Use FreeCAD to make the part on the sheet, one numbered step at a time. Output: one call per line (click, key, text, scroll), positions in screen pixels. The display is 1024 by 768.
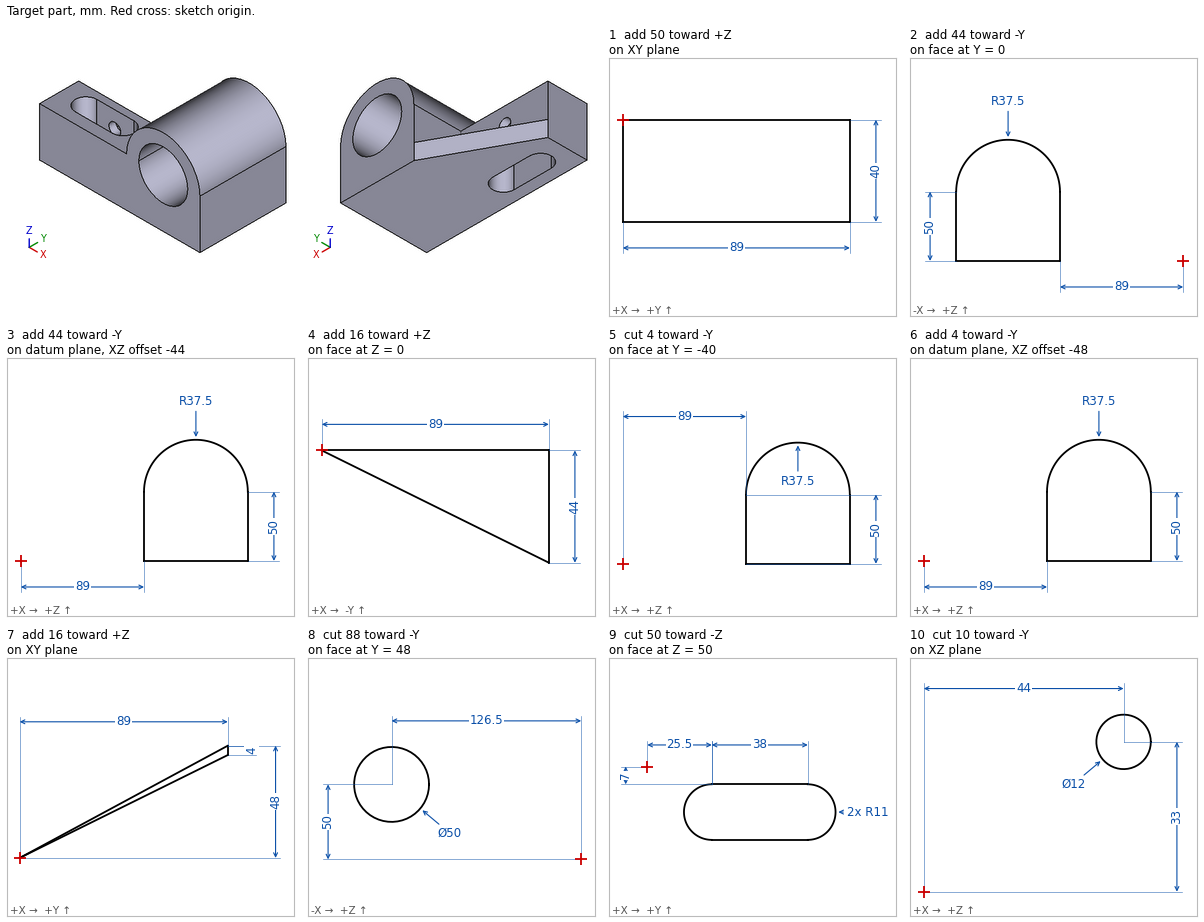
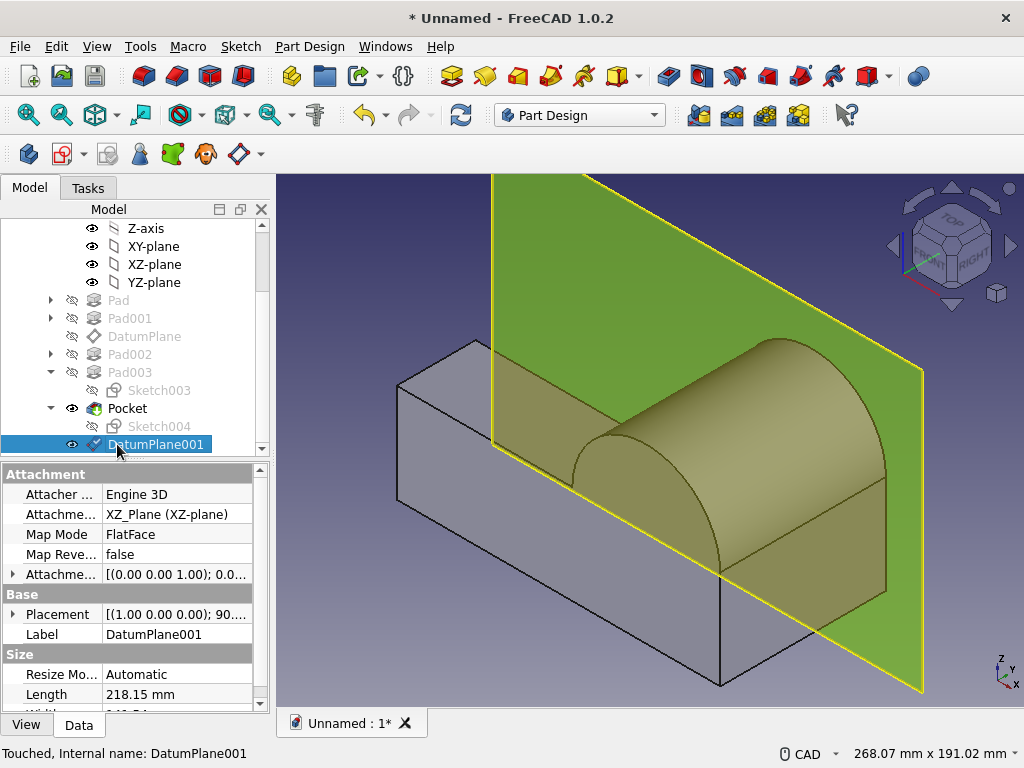
click(62, 154)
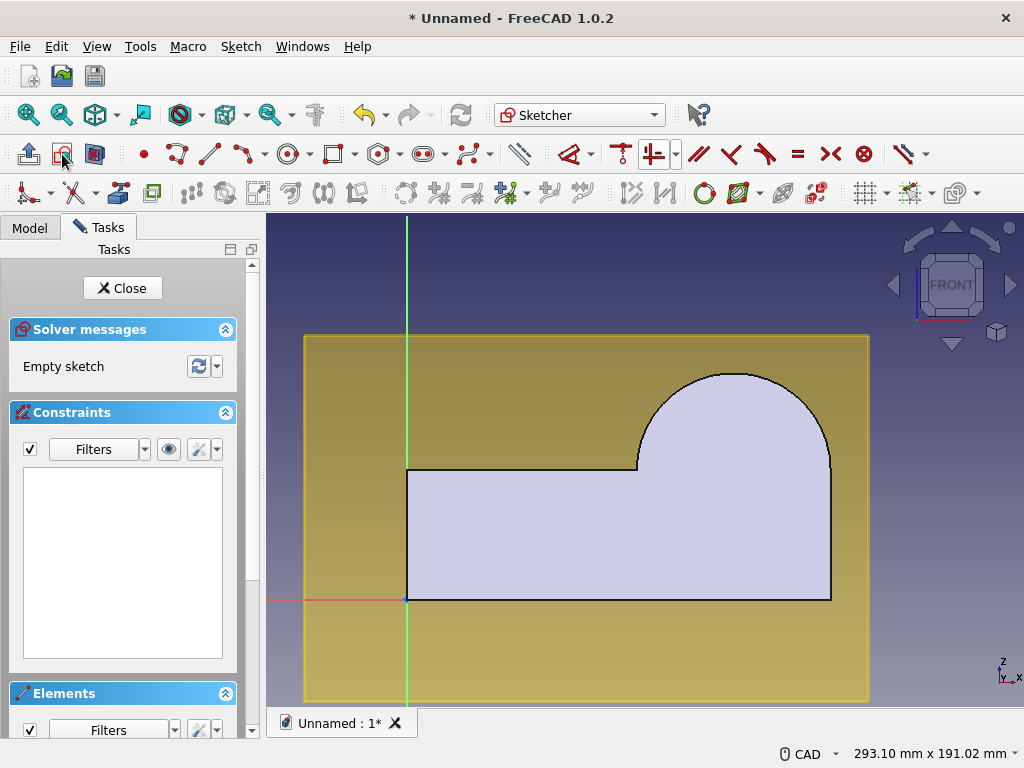
click(95, 154)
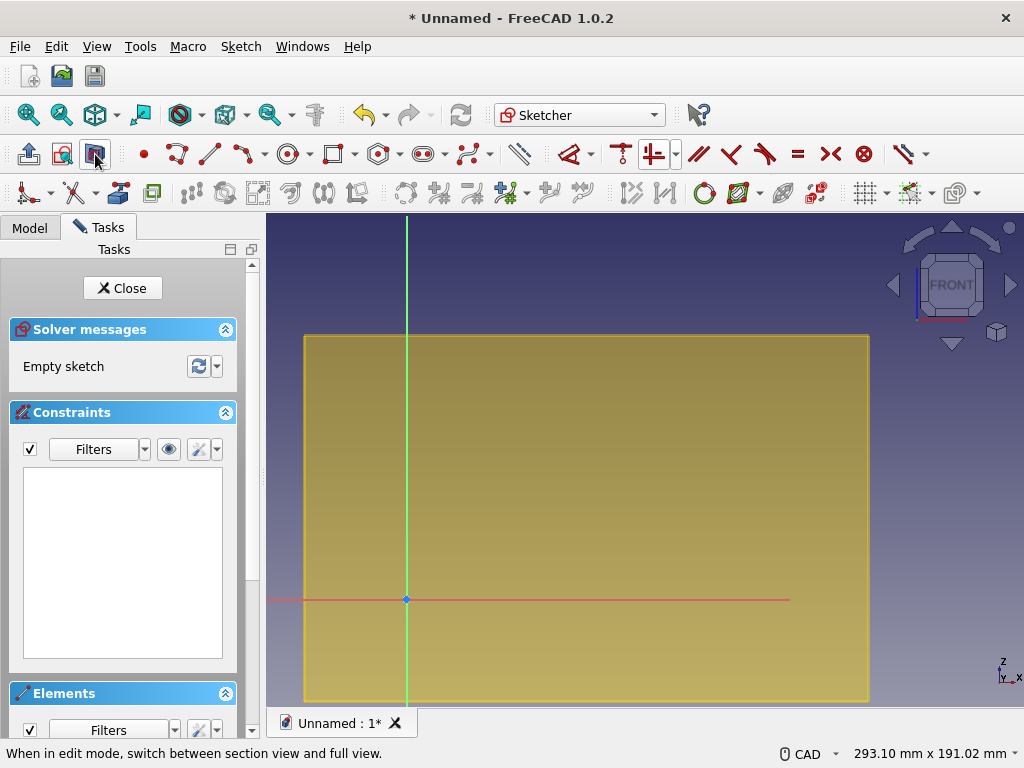
click(177, 154)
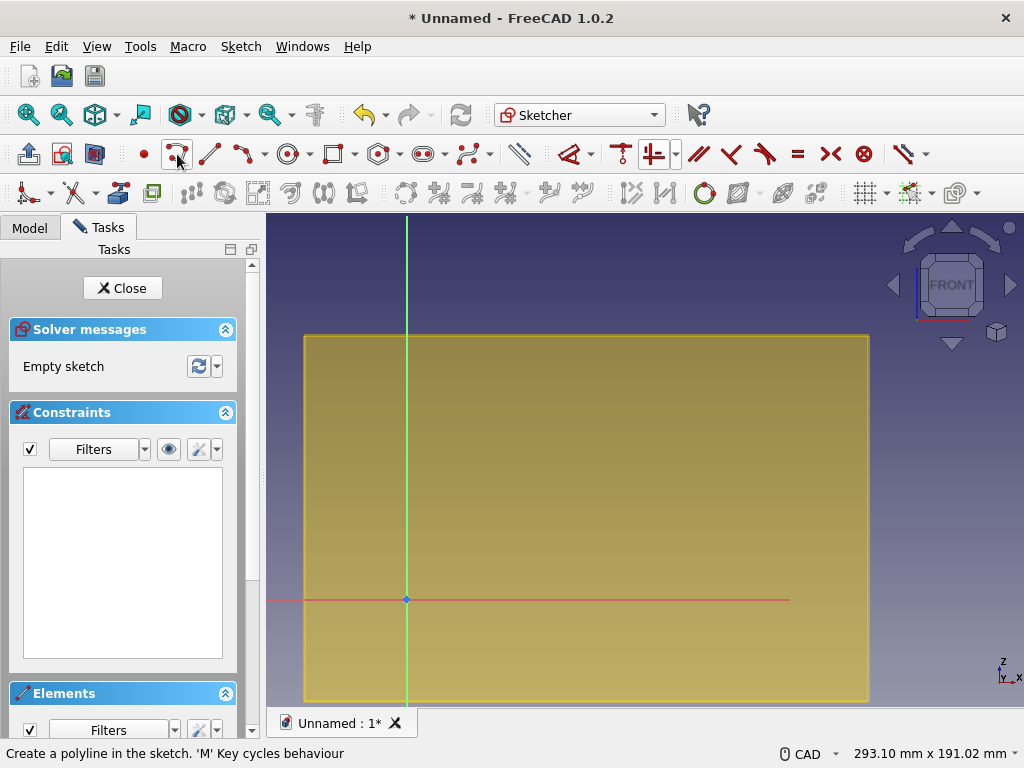
click(831, 470)
click(831, 600)
click(637, 591)
click(637, 470)
right_click(637, 470)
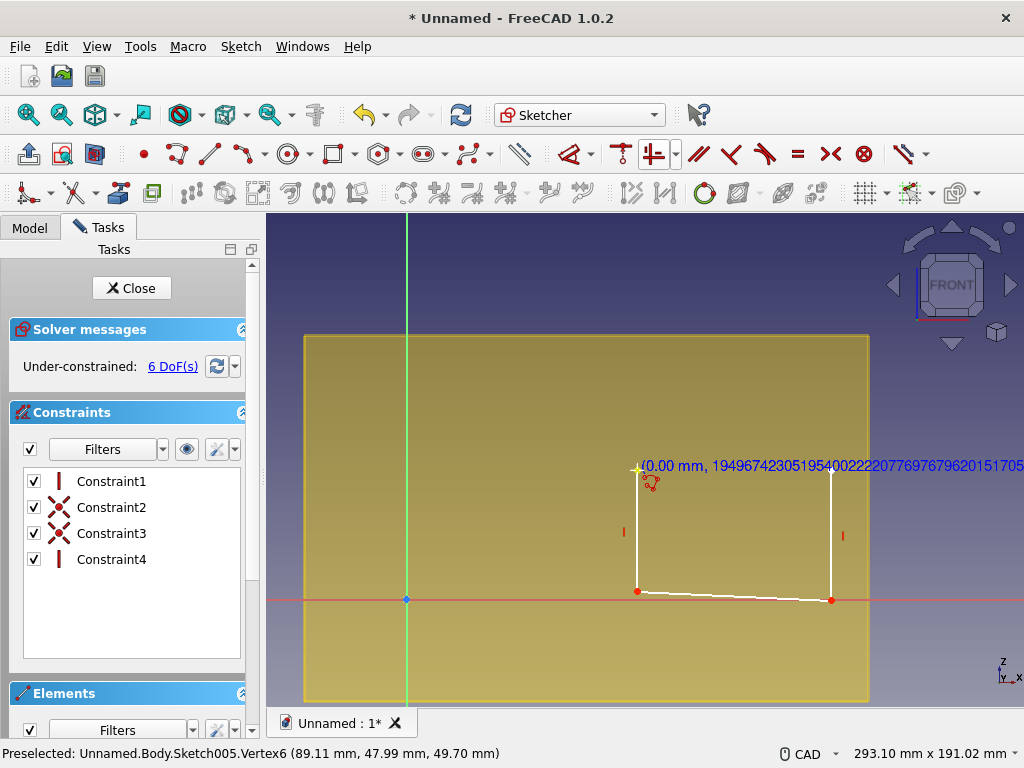
click(242, 154)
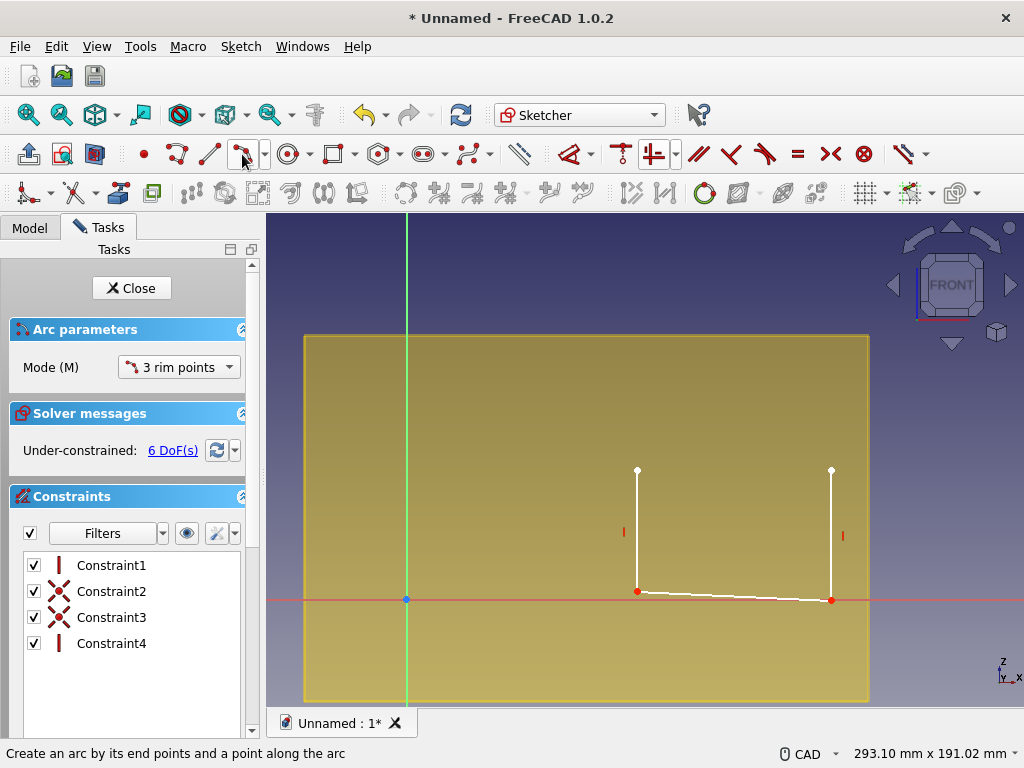
click(637, 471)
click(831, 471)
click(734, 373)
key(Escape)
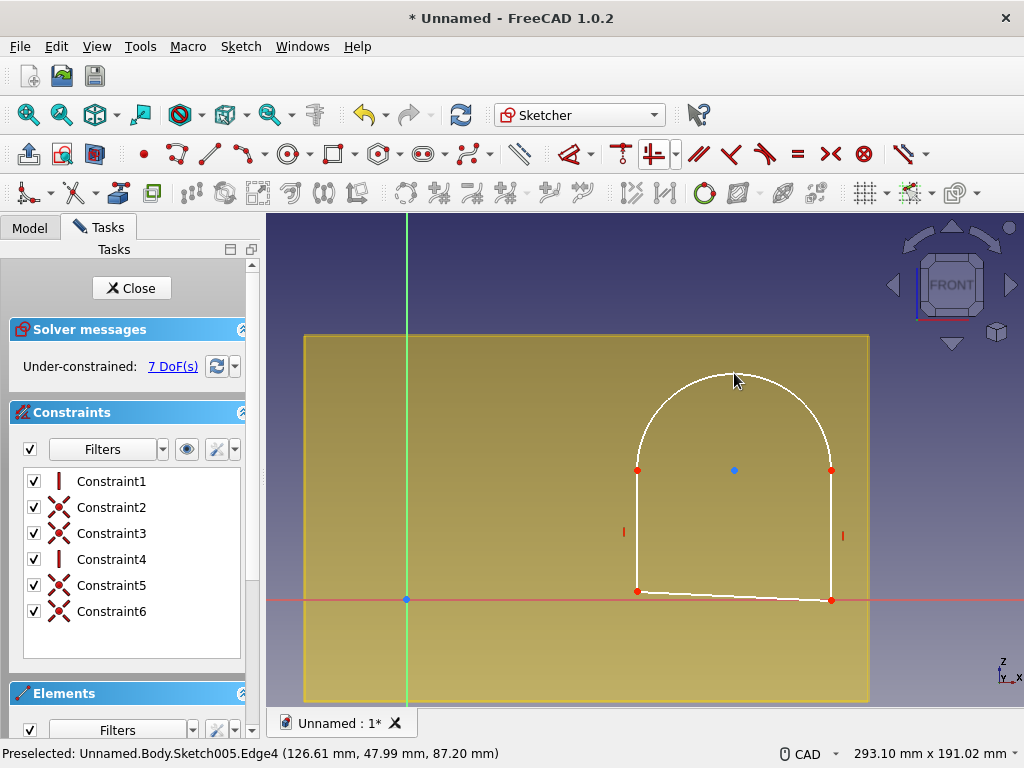
click(831, 510)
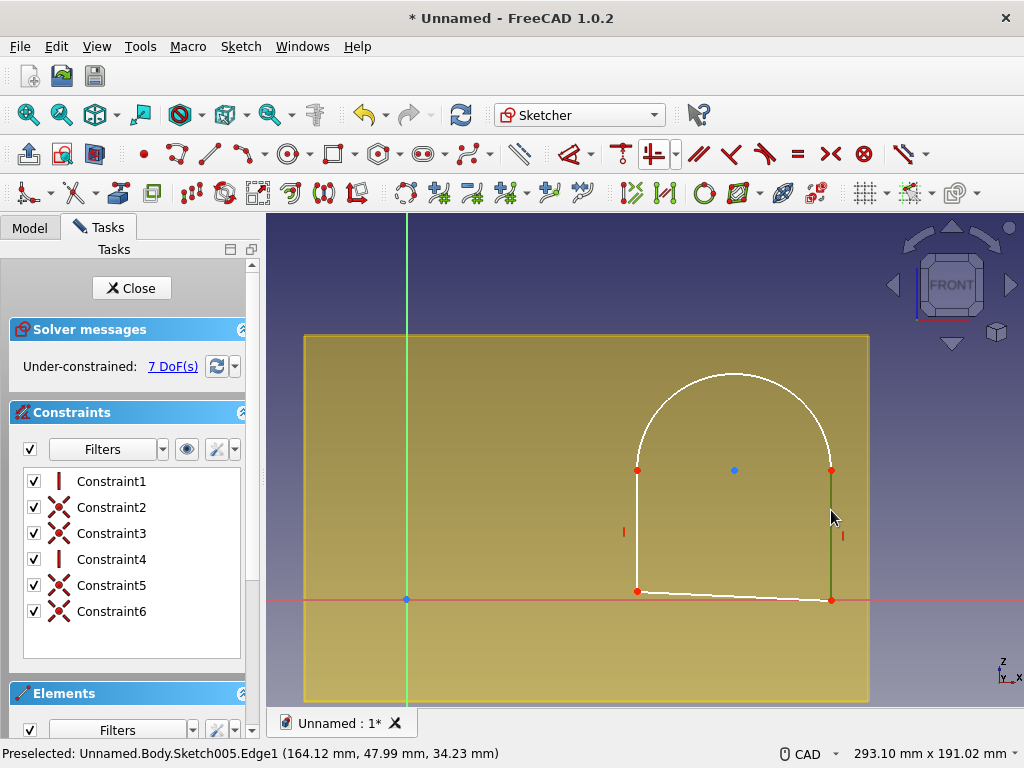
click(791, 393)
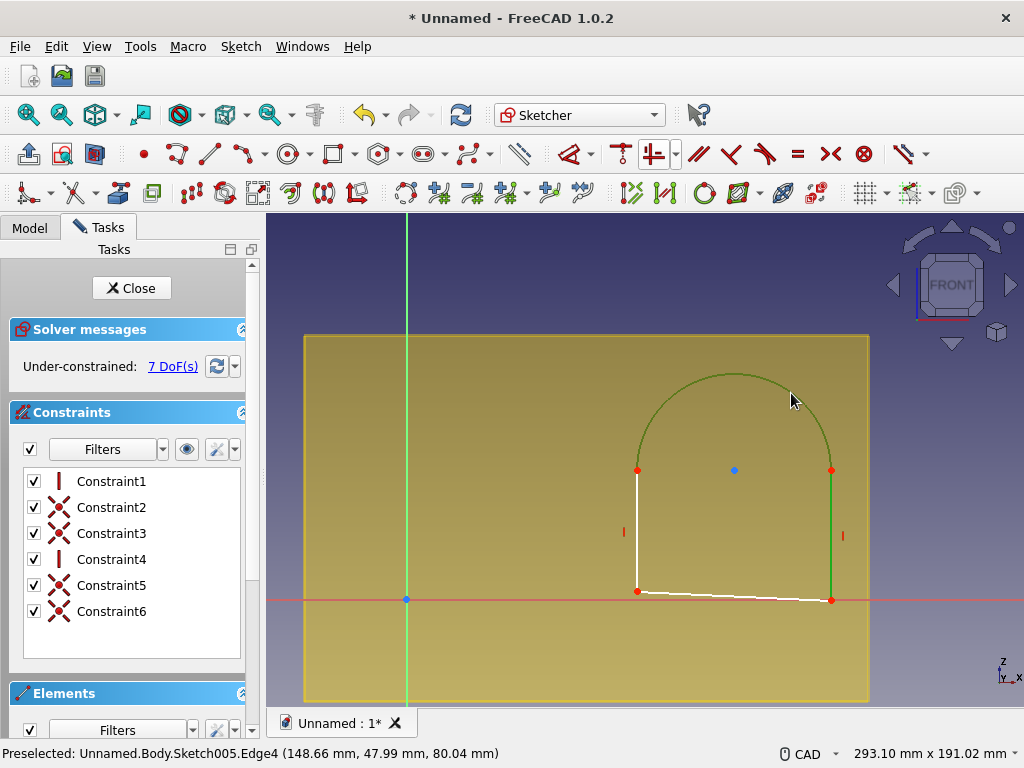
click(765, 154)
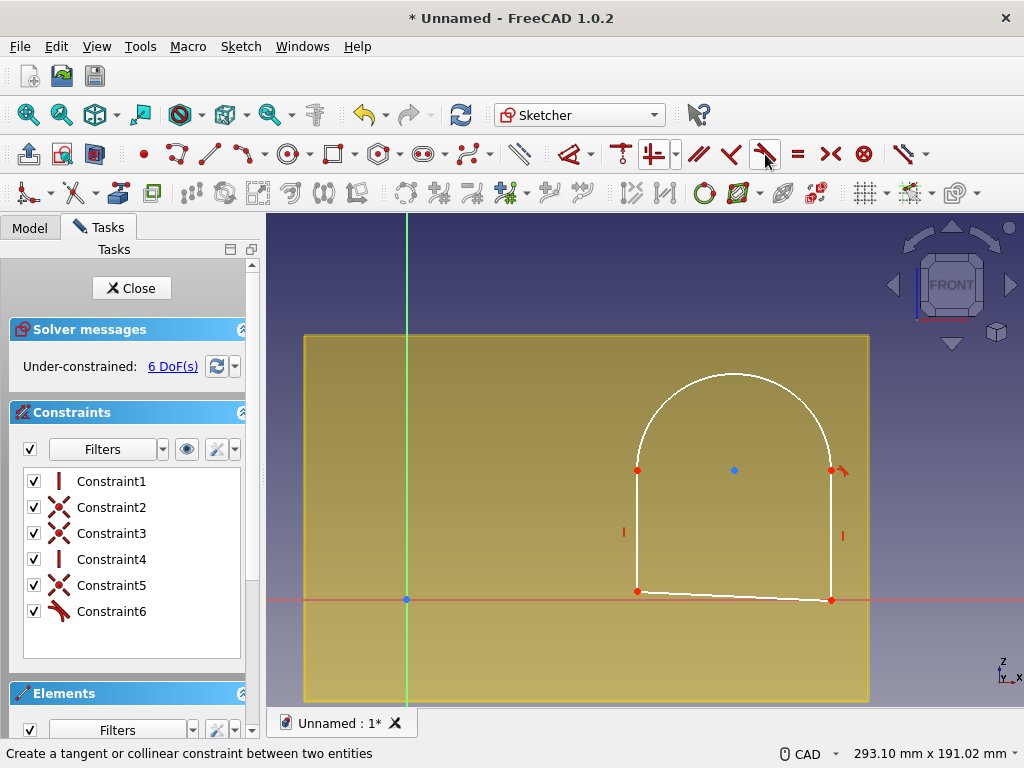
click(637, 556)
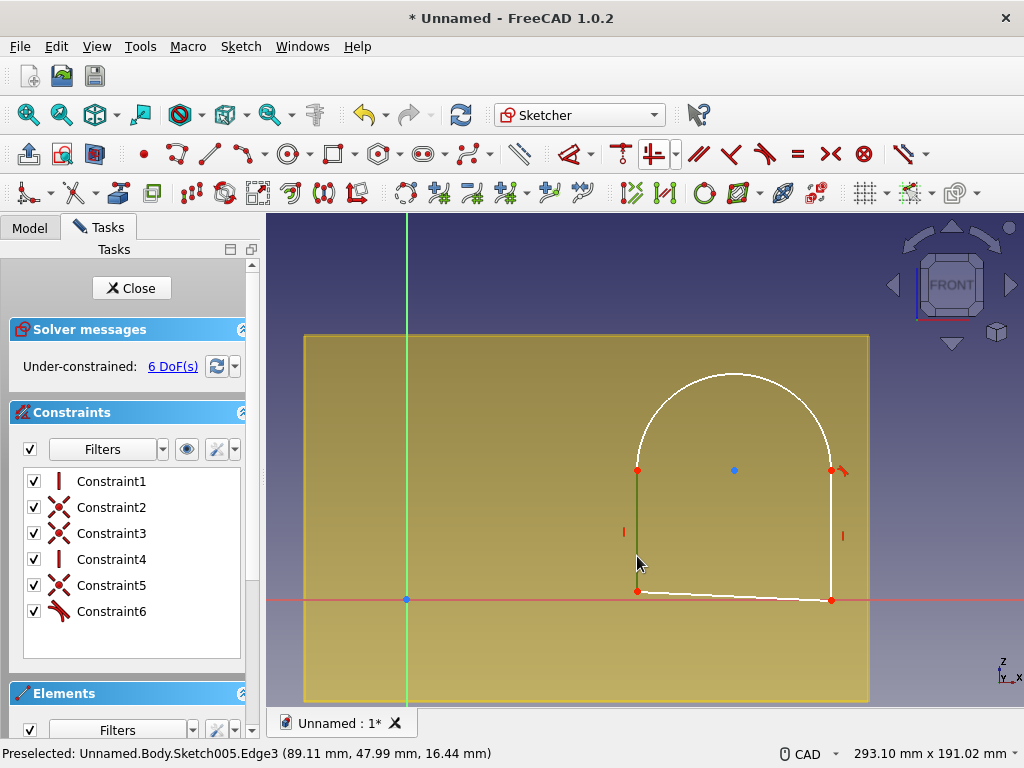
click(791, 393)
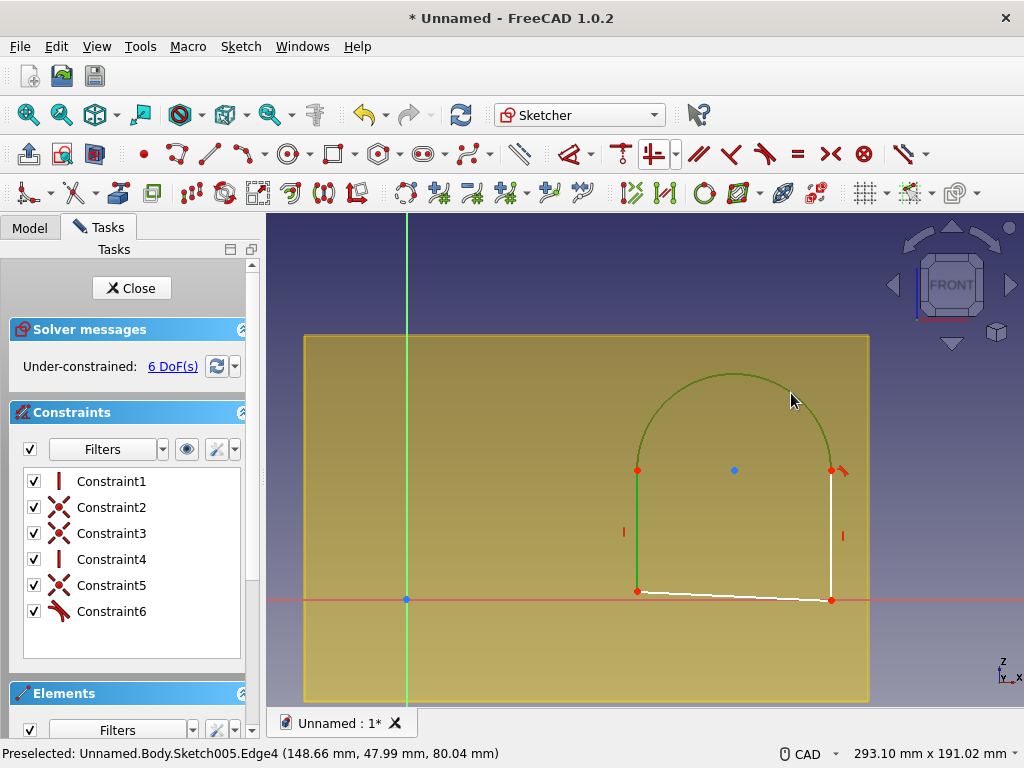
click(765, 154)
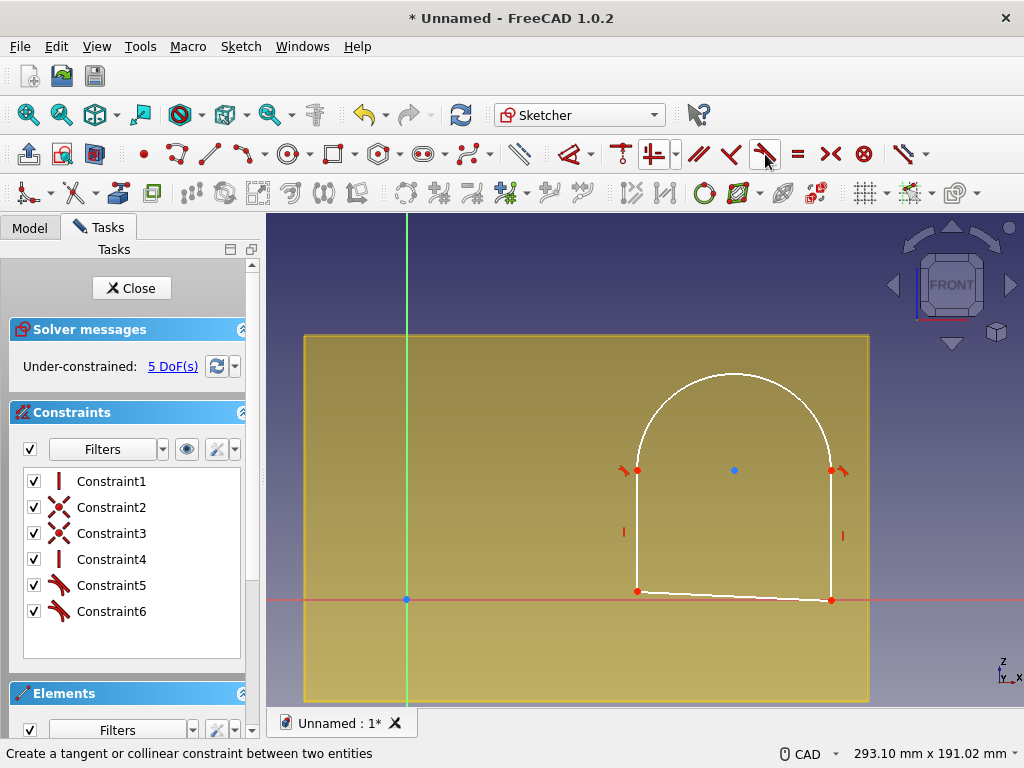
click(773, 598)